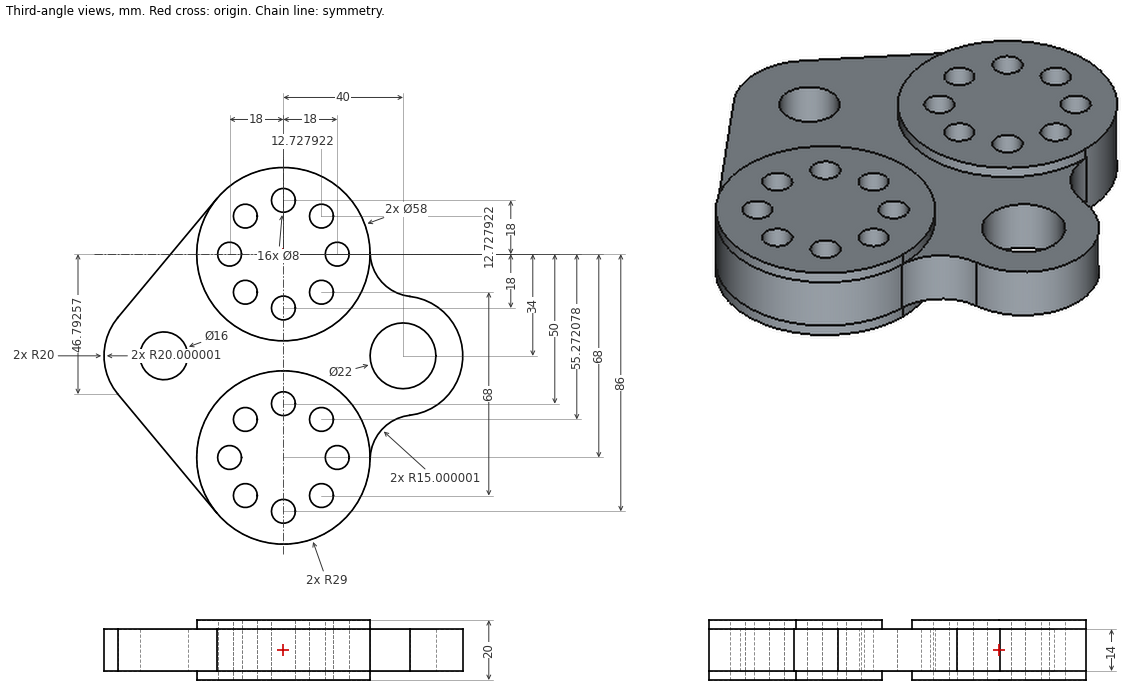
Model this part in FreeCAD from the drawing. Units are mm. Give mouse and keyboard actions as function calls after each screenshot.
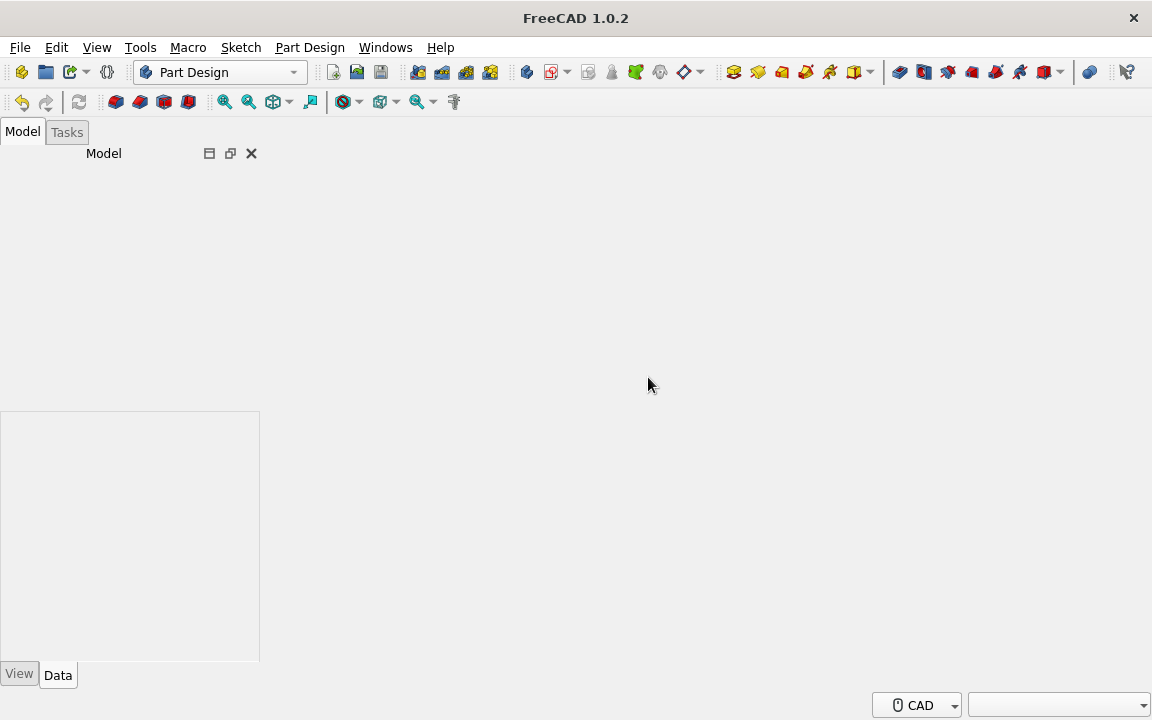
click(334, 72)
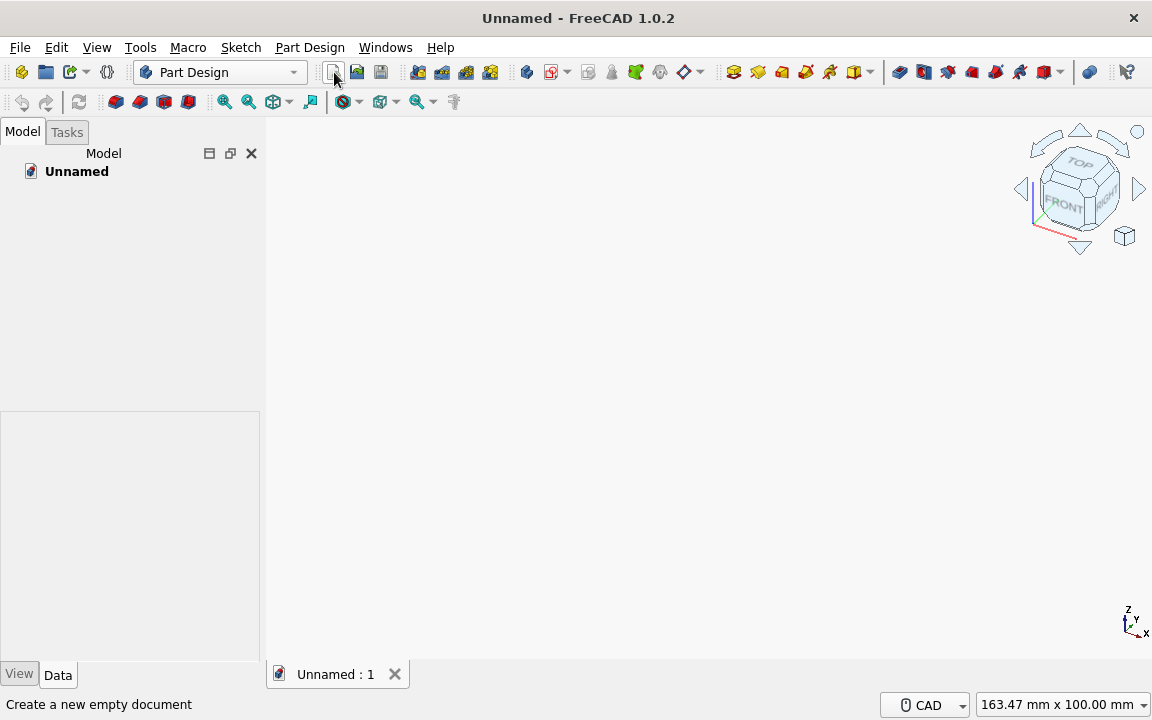
click(552, 72)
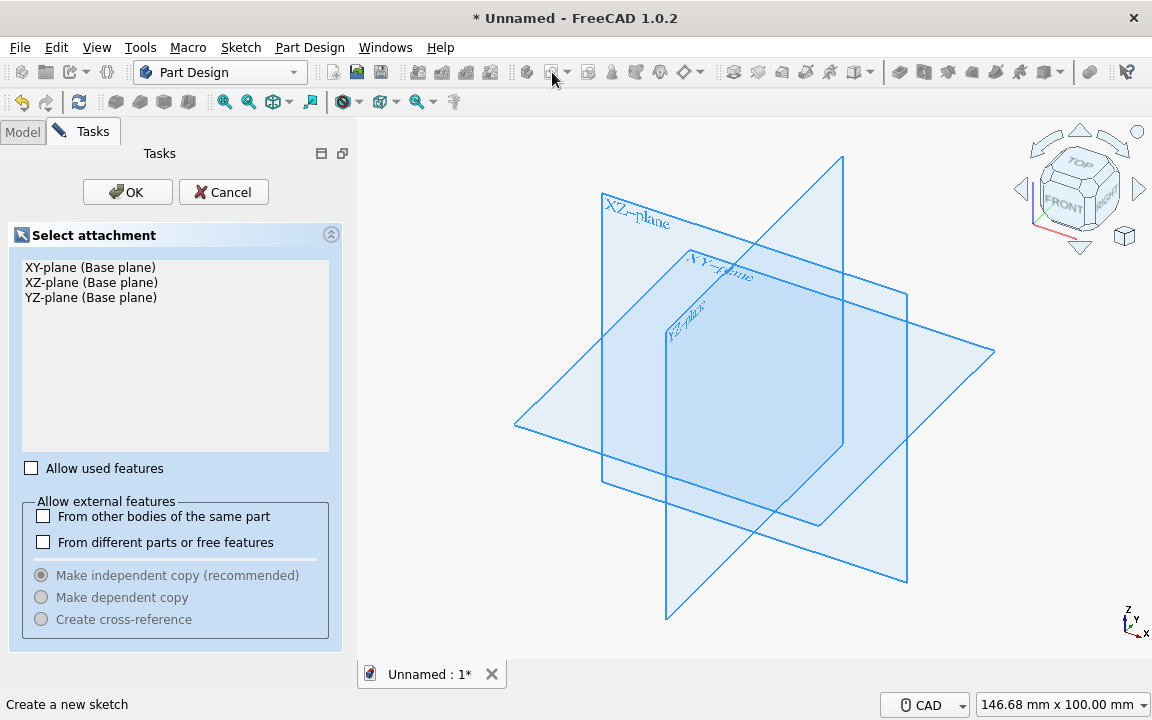
click(82, 268)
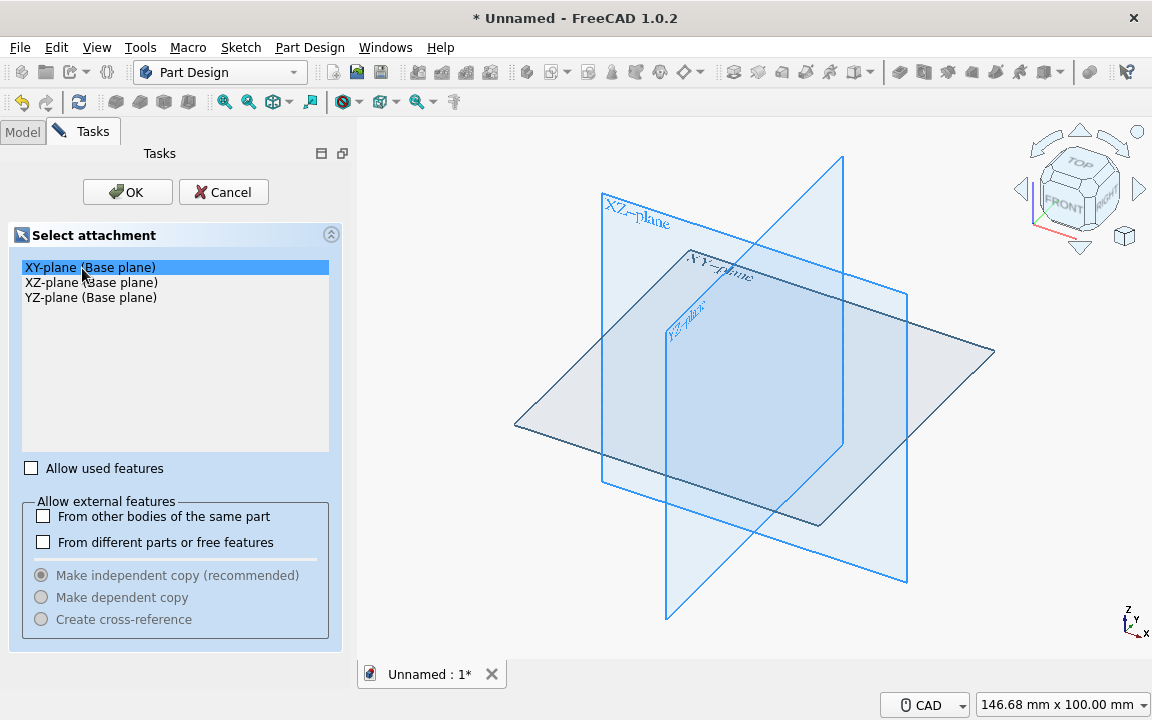
click(128, 192)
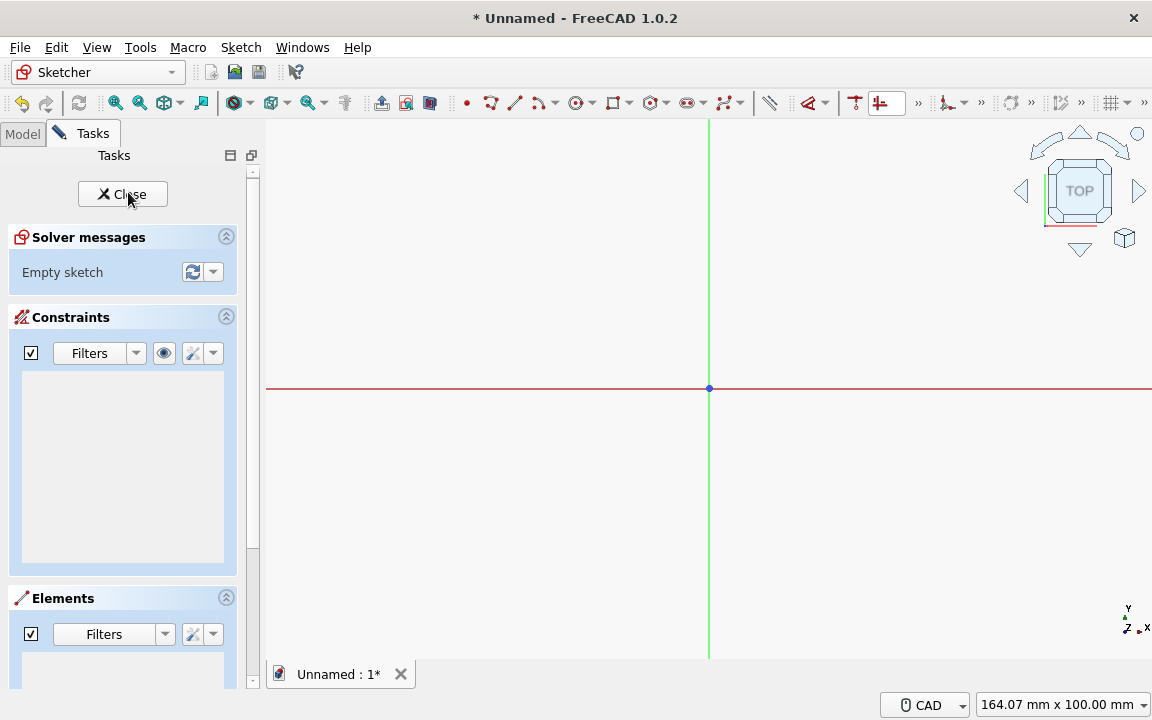
scroll(557, 166, down, 3)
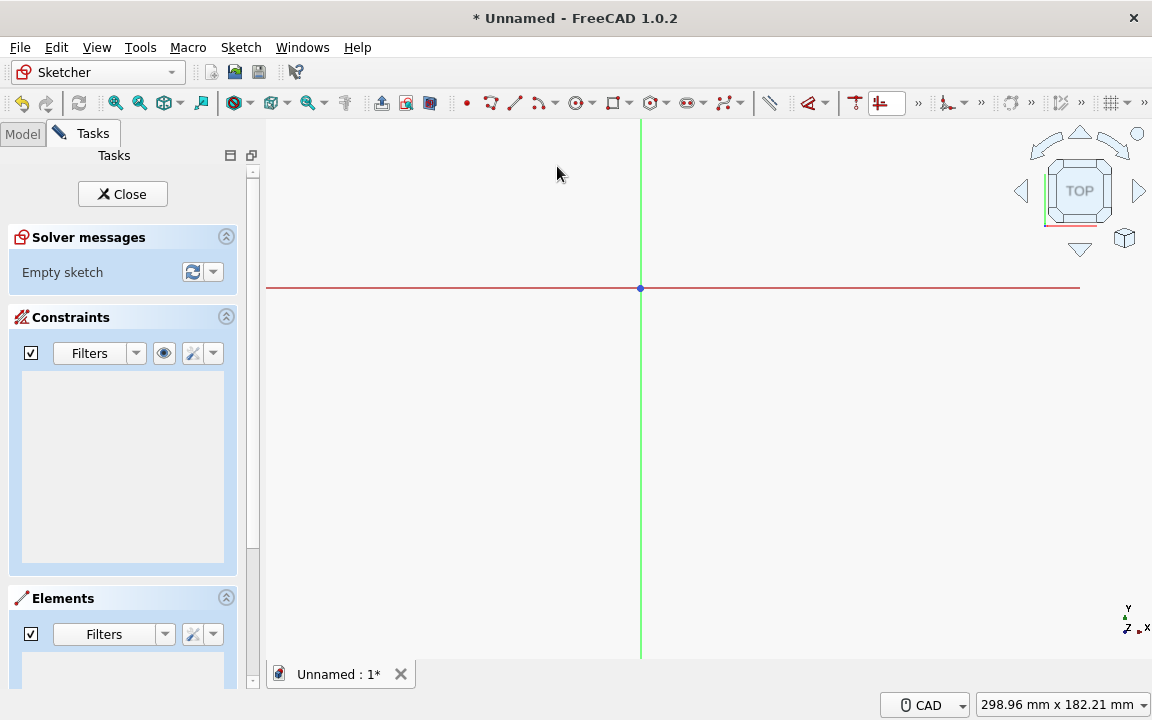
key(g)
key(l)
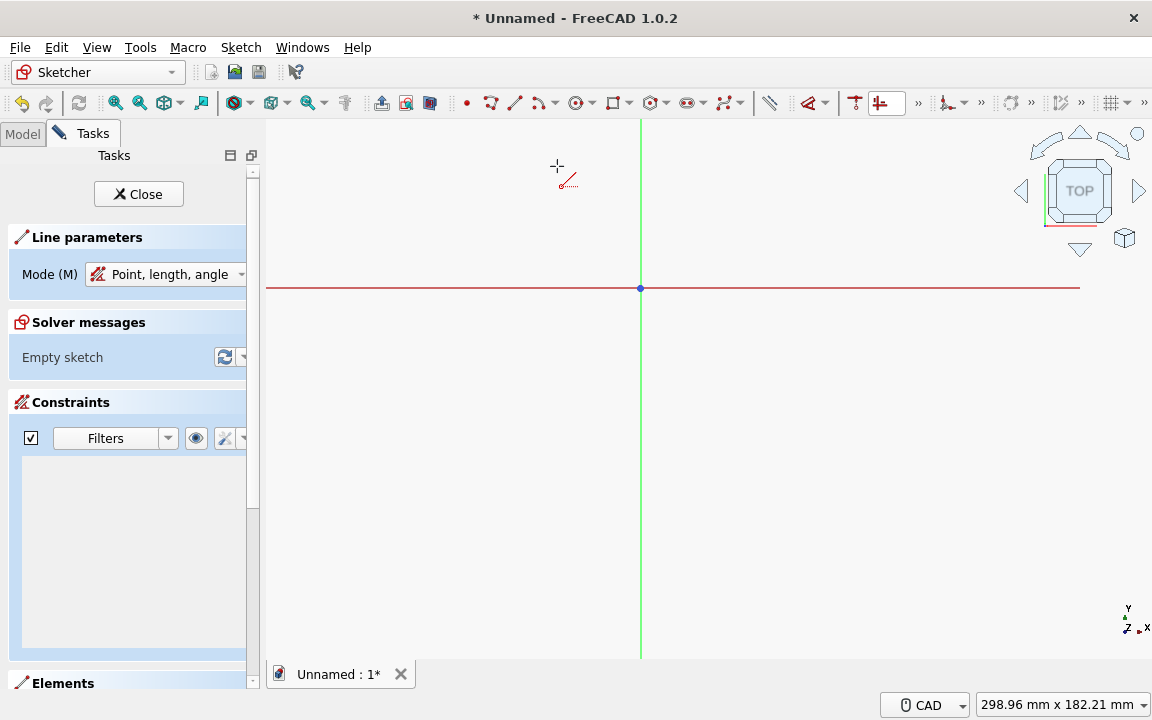
click(575, 233)
click(476, 351)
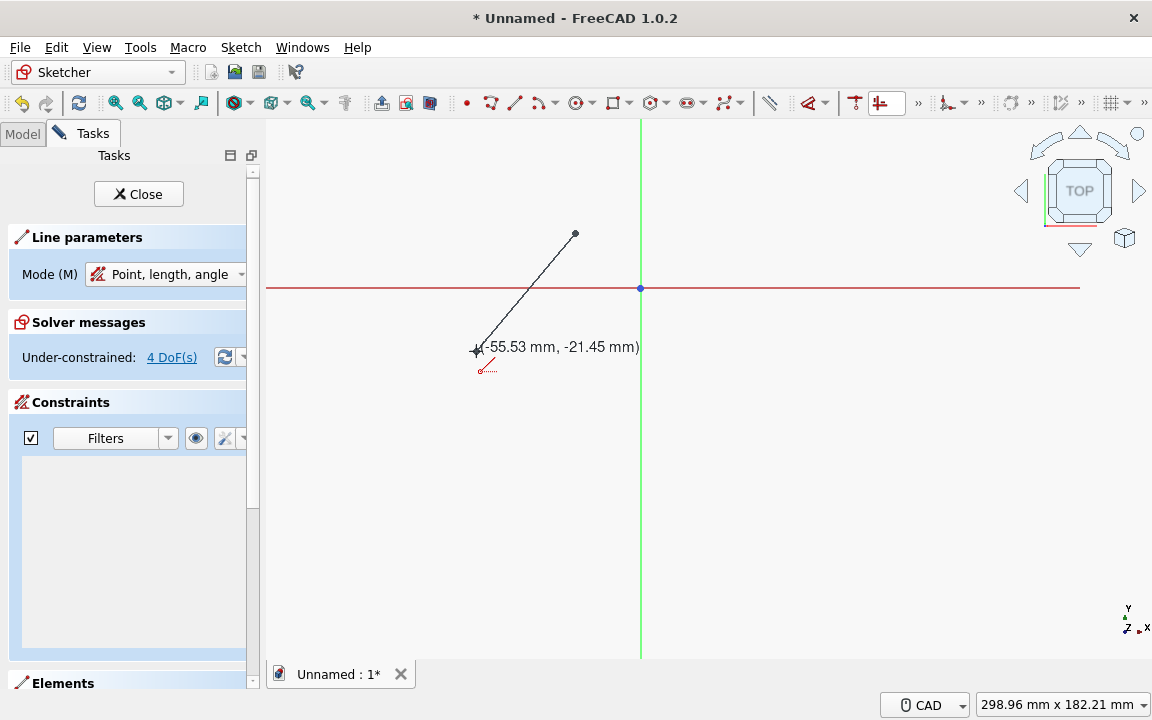
click(476, 427)
click(575, 545)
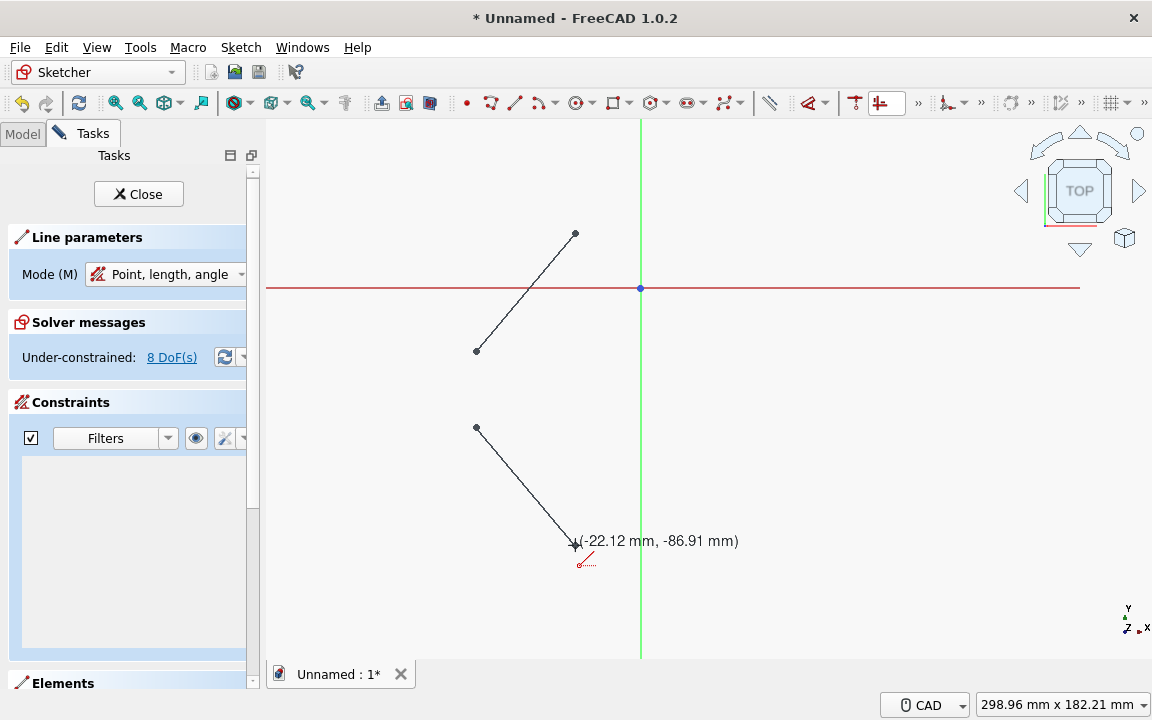
key(g)
key(3)
key(a)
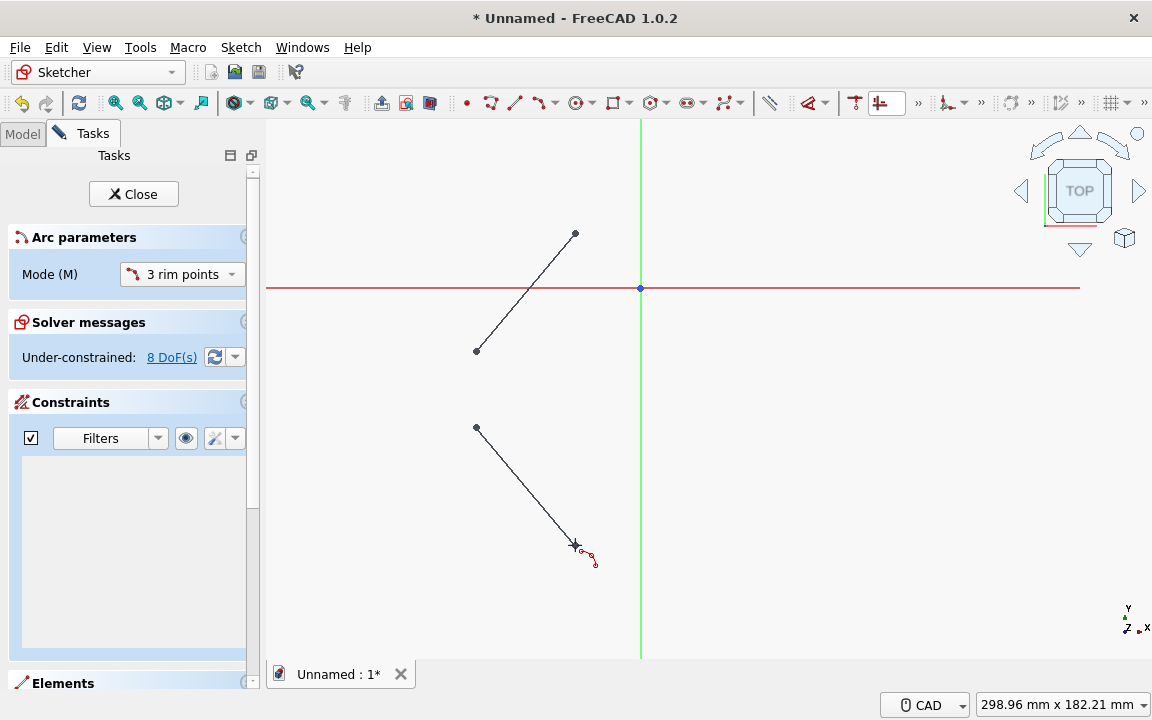
click(476, 352)
click(476, 428)
click(463, 389)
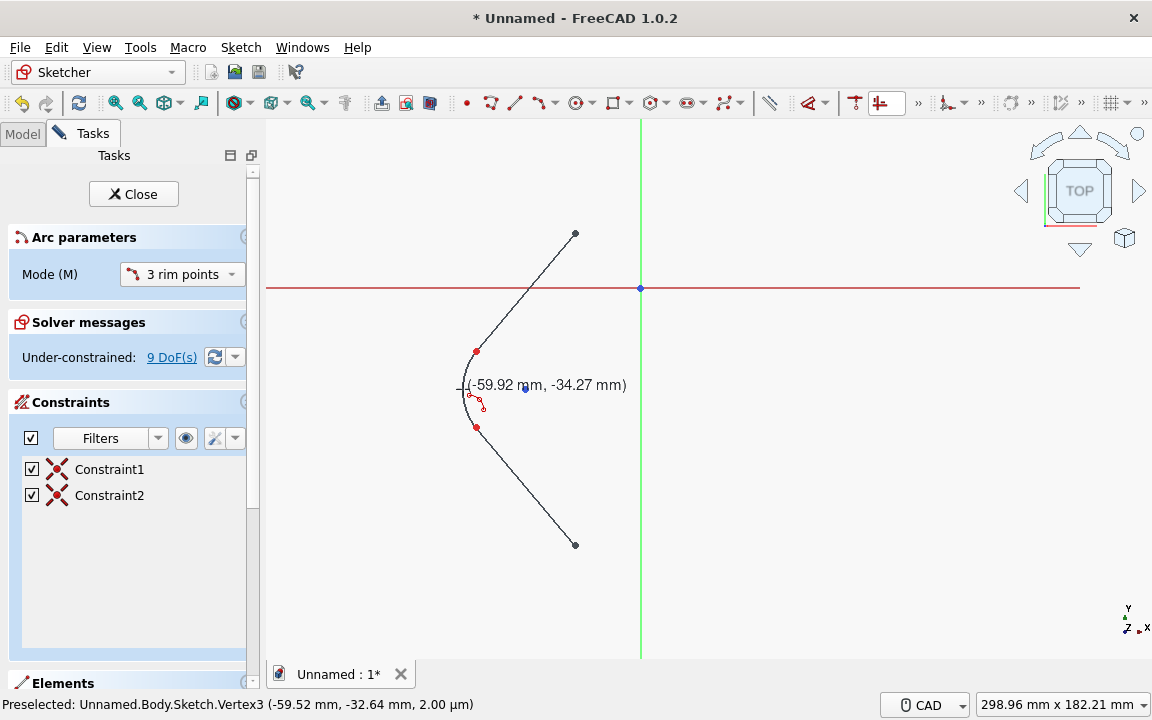
click(575, 546)
click(726, 491)
click(669, 571)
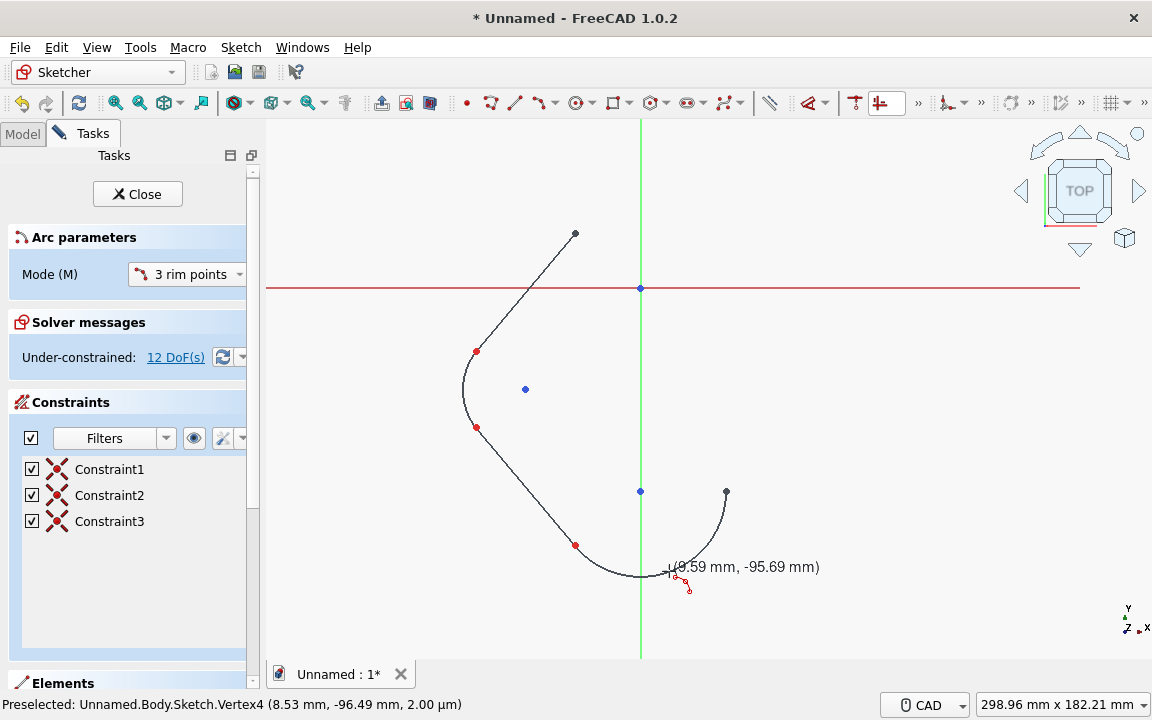
click(726, 492)
click(766, 448)